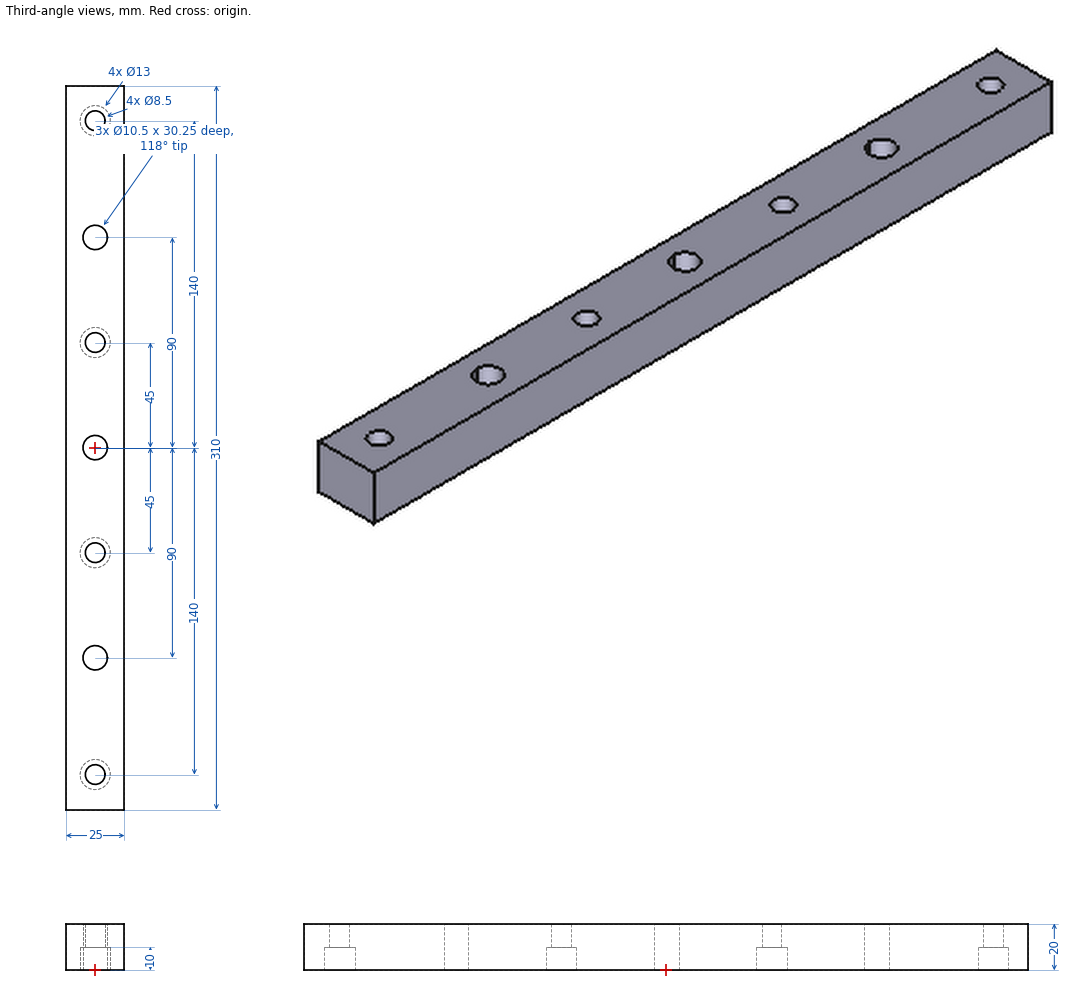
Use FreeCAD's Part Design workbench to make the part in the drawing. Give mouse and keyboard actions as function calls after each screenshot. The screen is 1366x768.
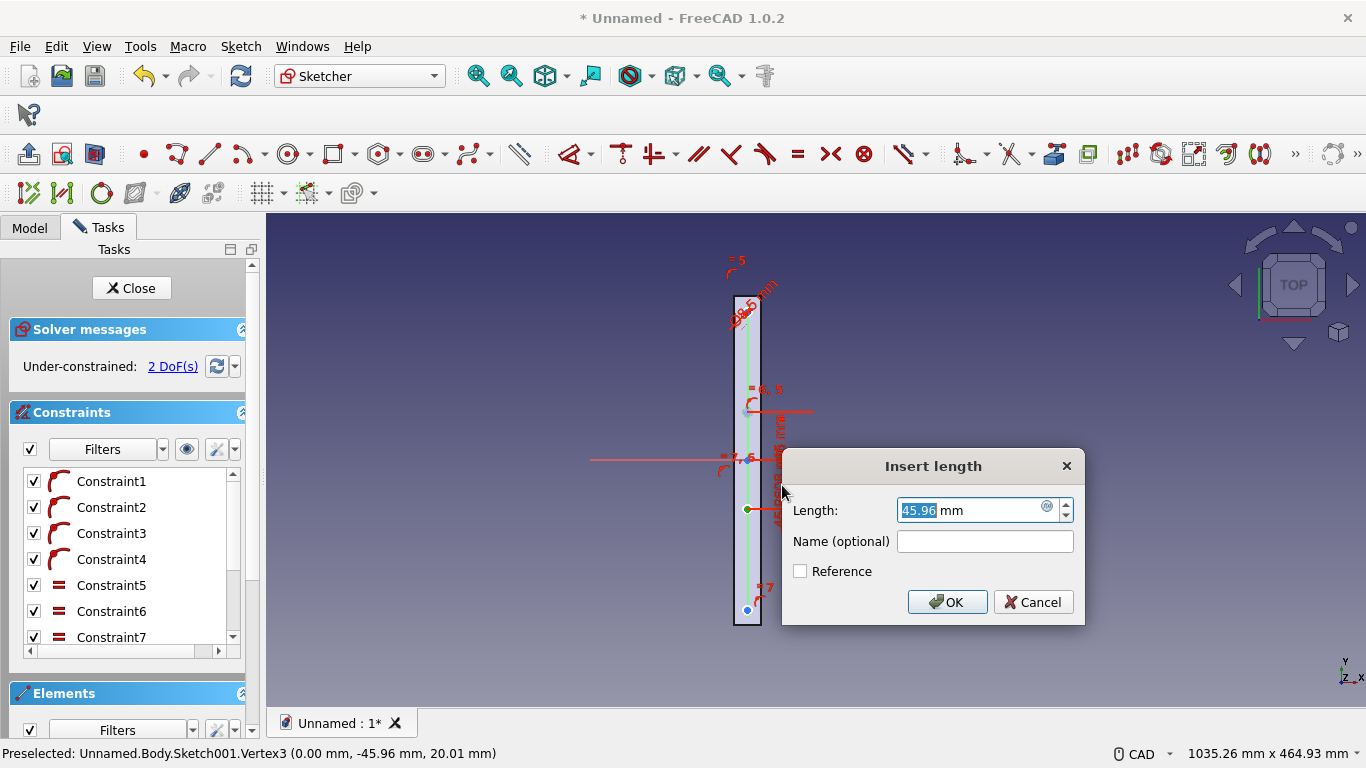
text(45)
key(Return)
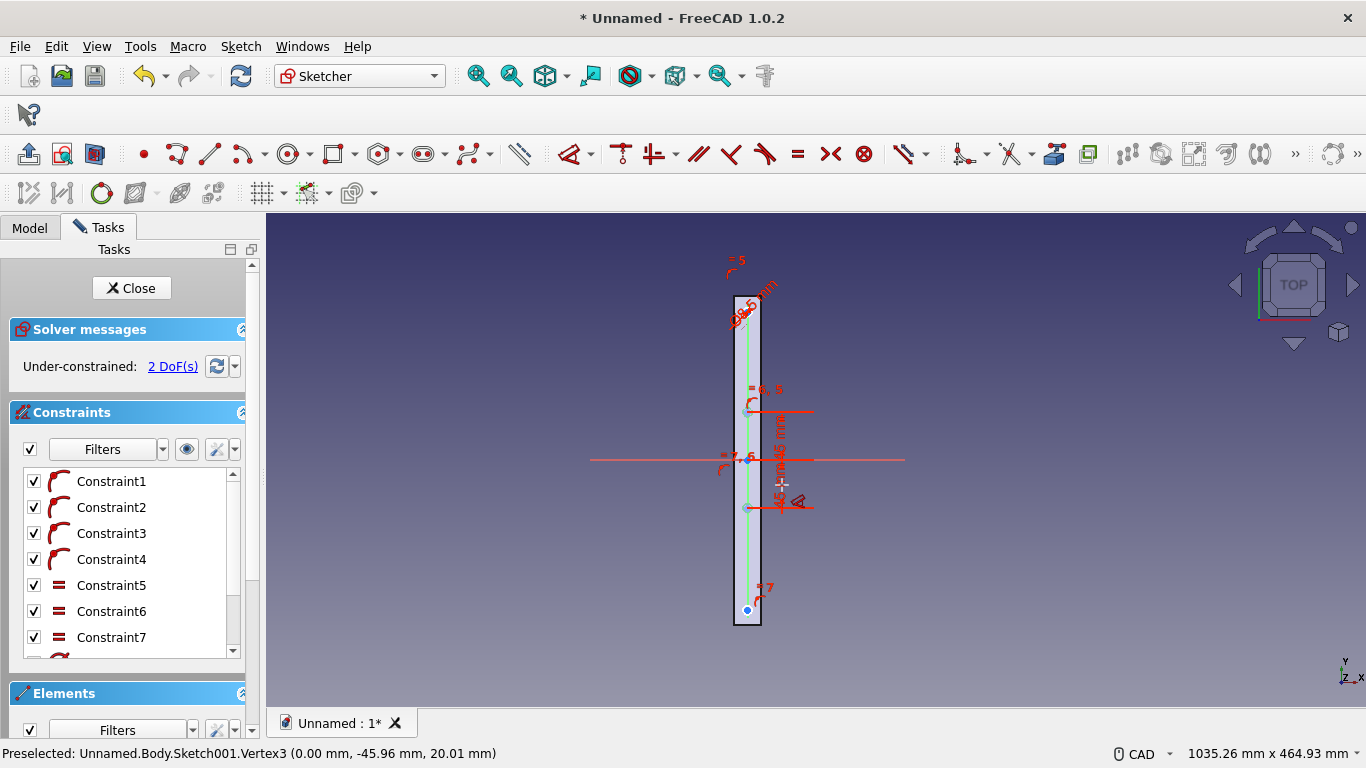
click(748, 312)
click(782, 386)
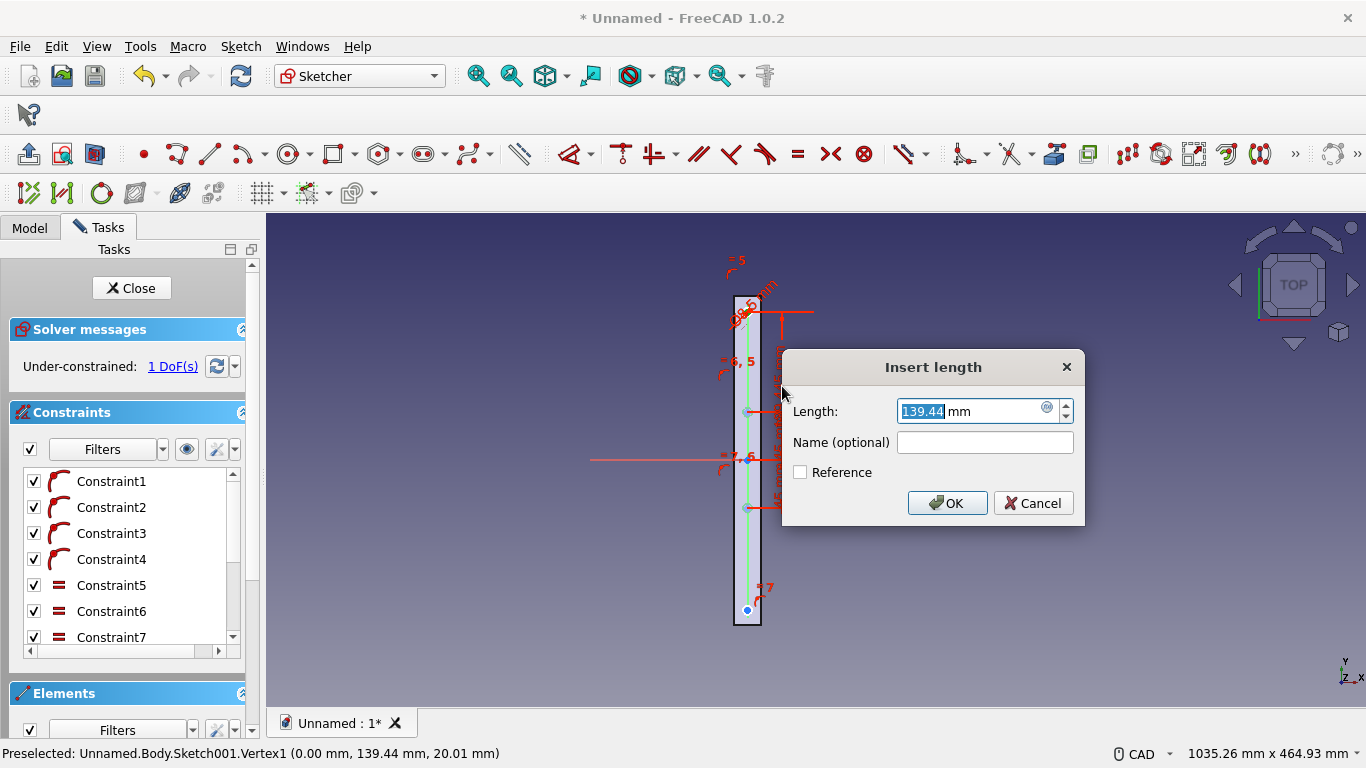
text(140)
key(Return)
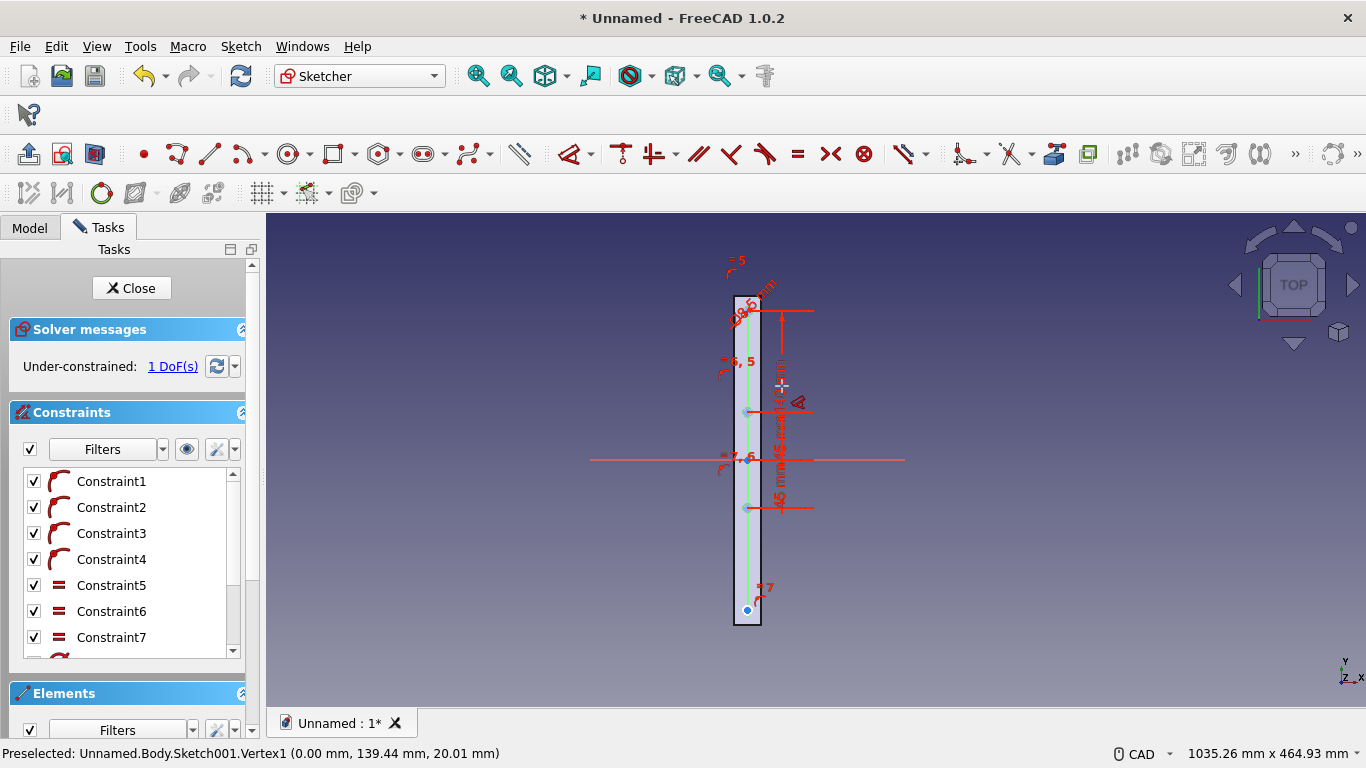
click(748, 610)
click(782, 535)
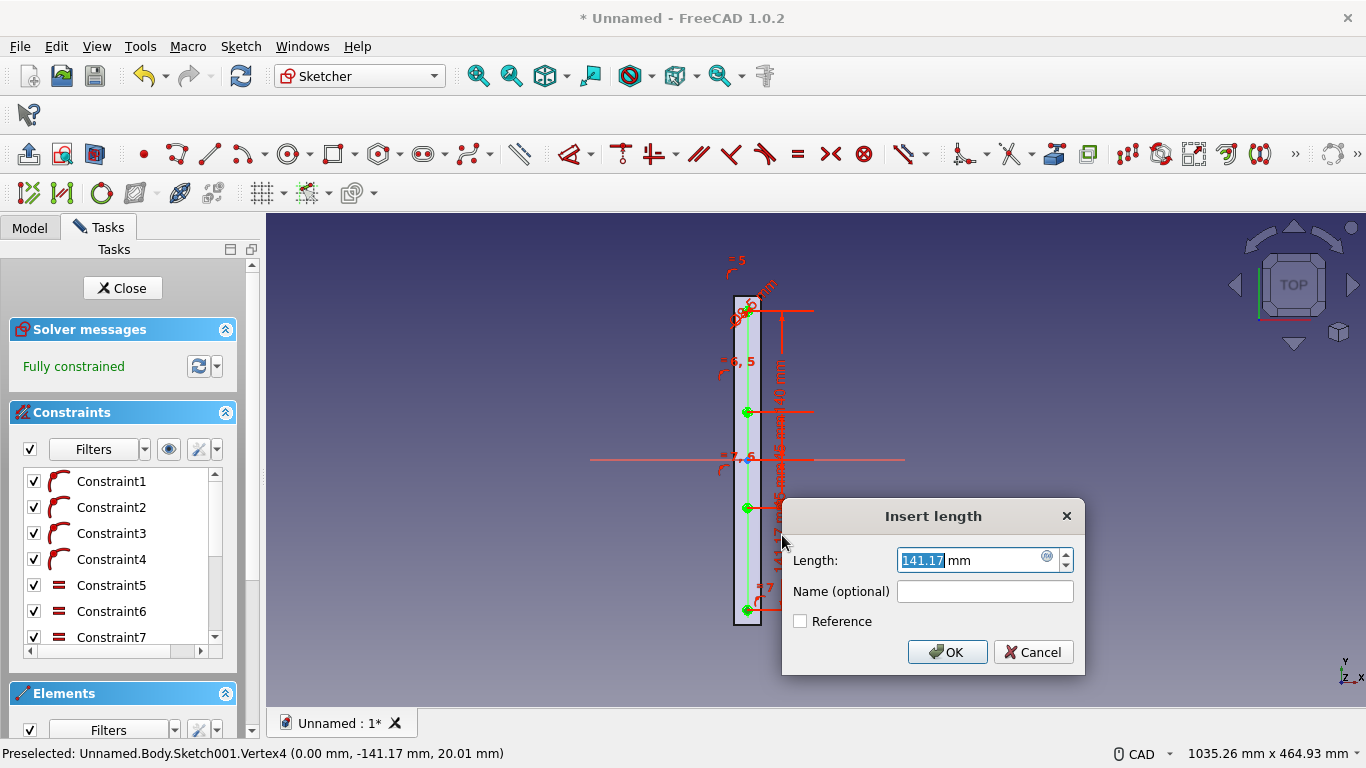
text(140)
key(Return)
key(Escape)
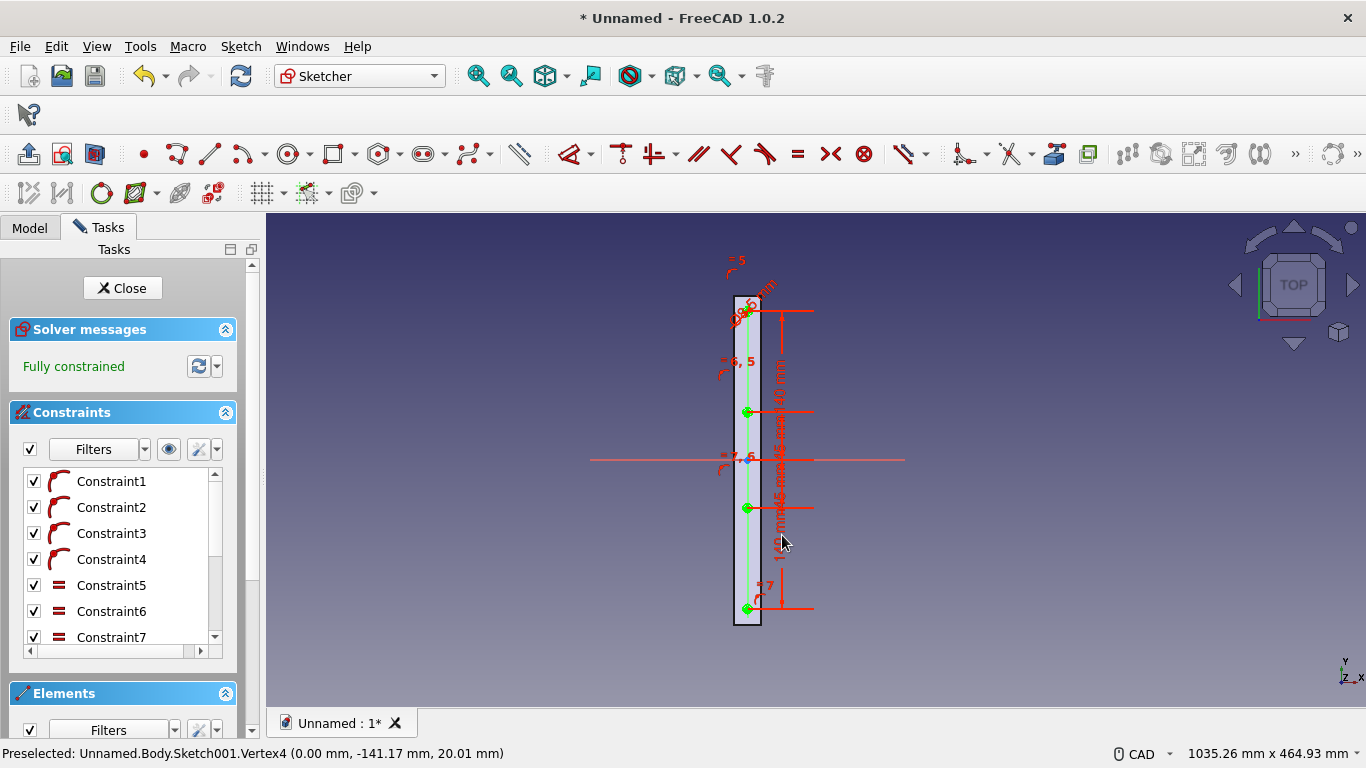
click(123, 288)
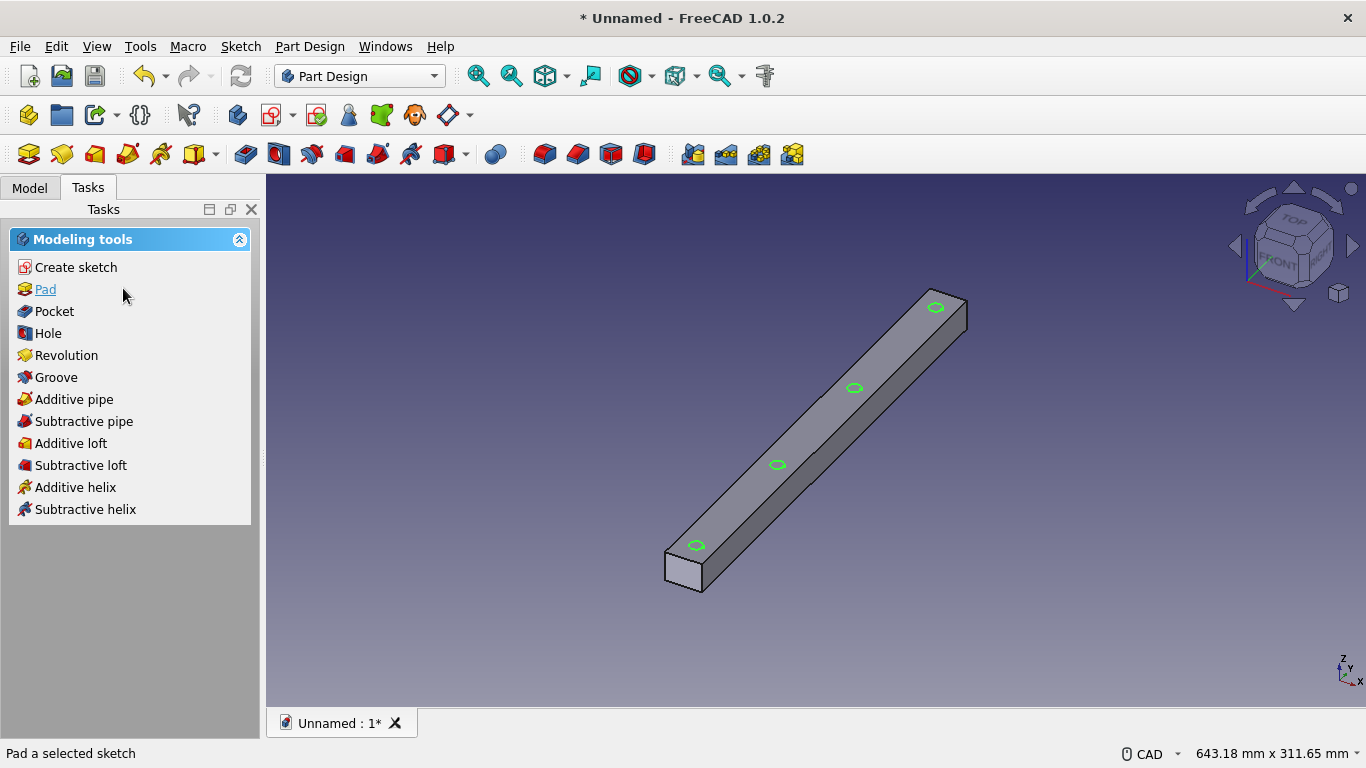
click(246, 154)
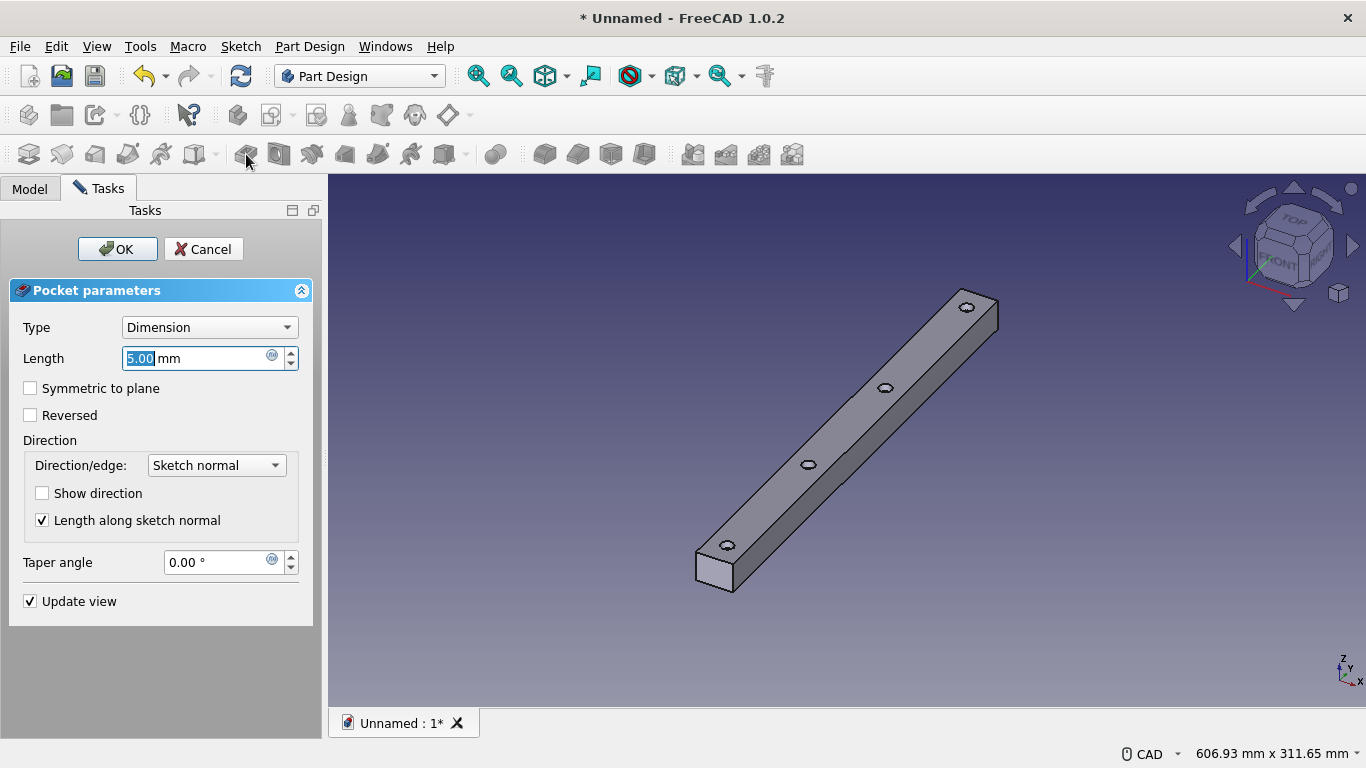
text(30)
key(Tab)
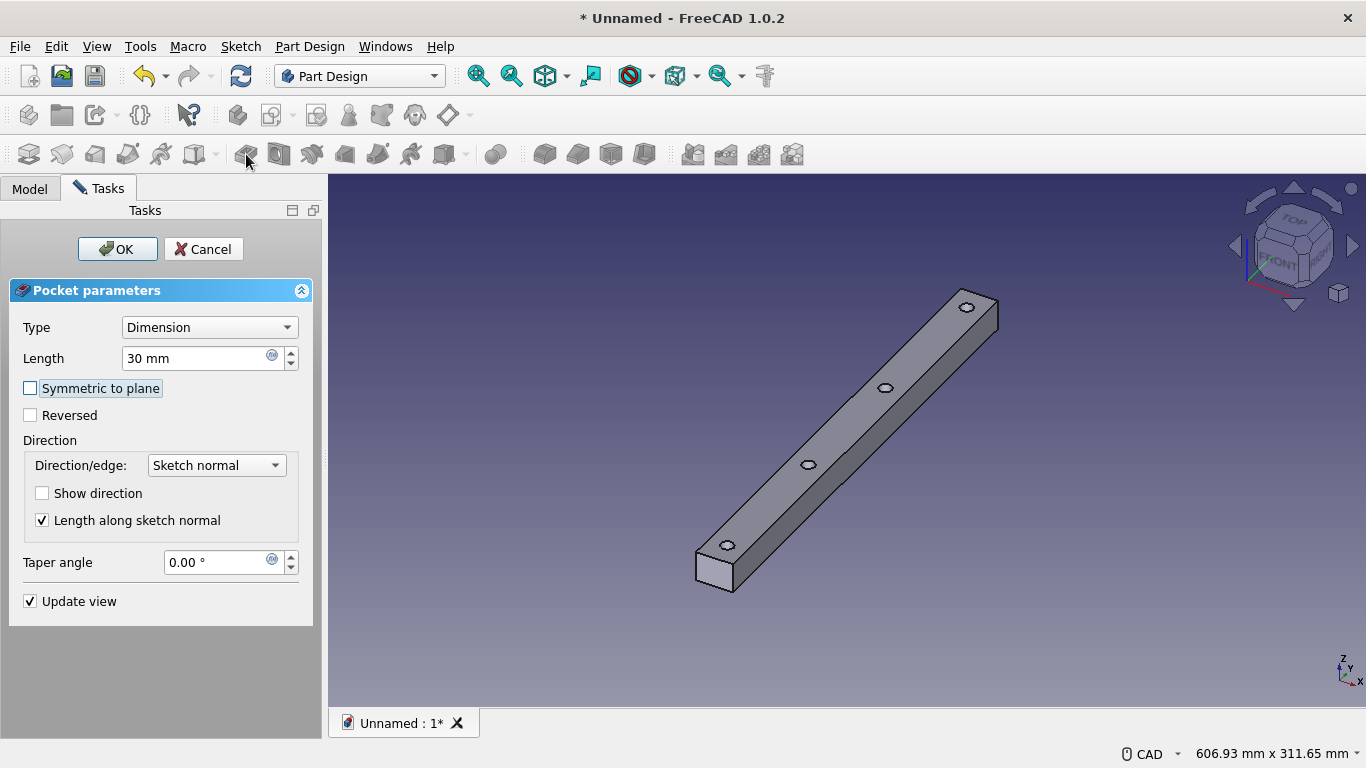
click(118, 249)